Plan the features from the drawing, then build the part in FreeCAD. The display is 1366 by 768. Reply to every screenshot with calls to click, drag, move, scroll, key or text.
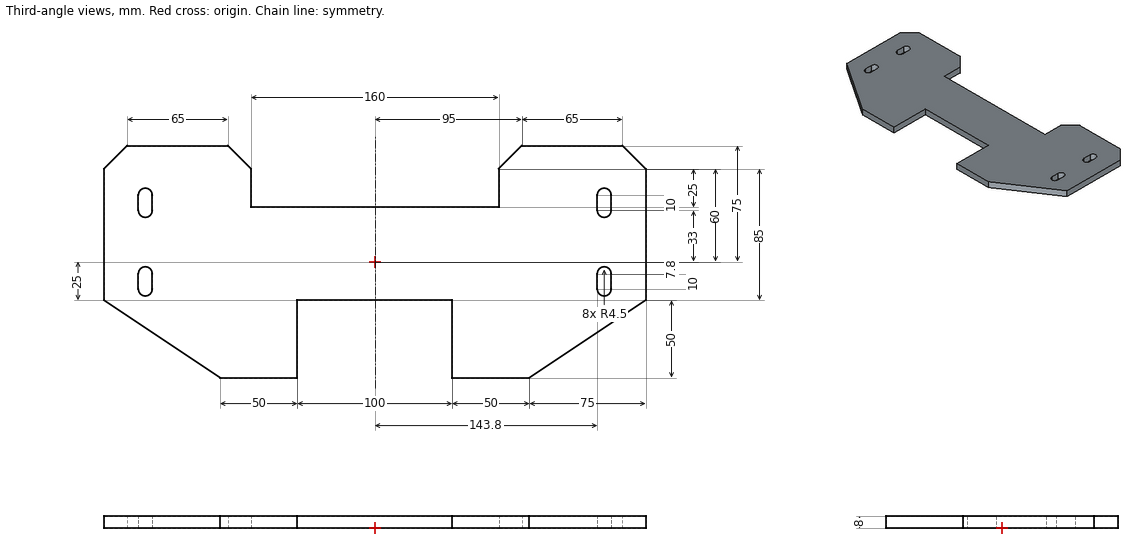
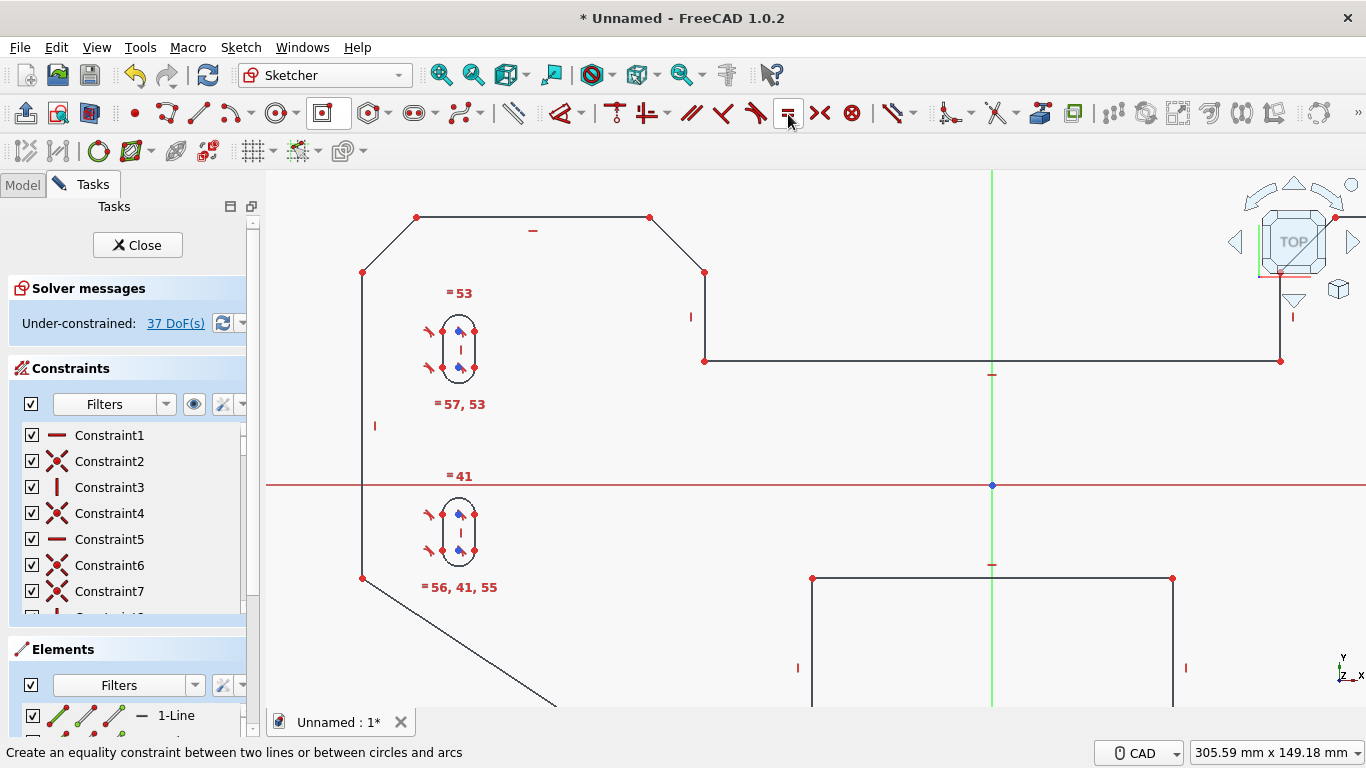
scroll(449, 381, down, 3)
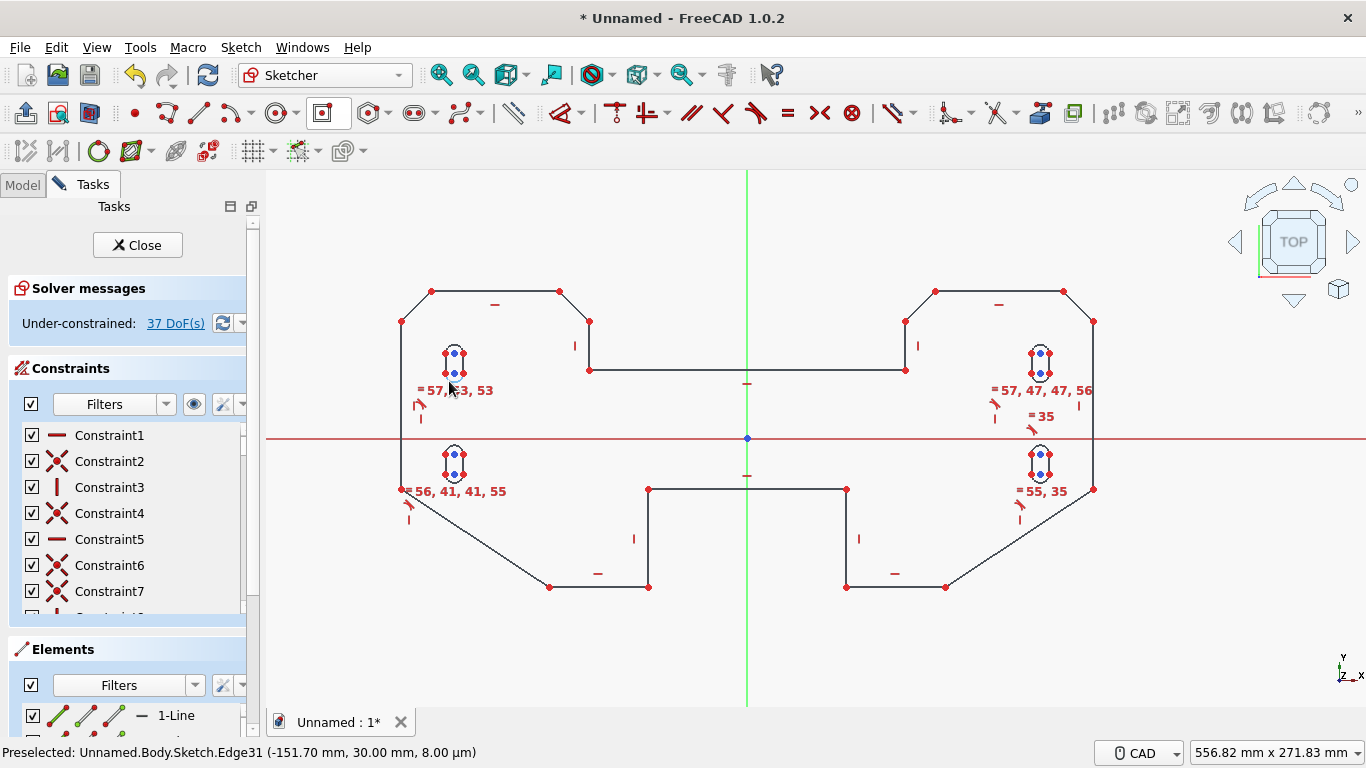
scroll(1040, 474, up, 2)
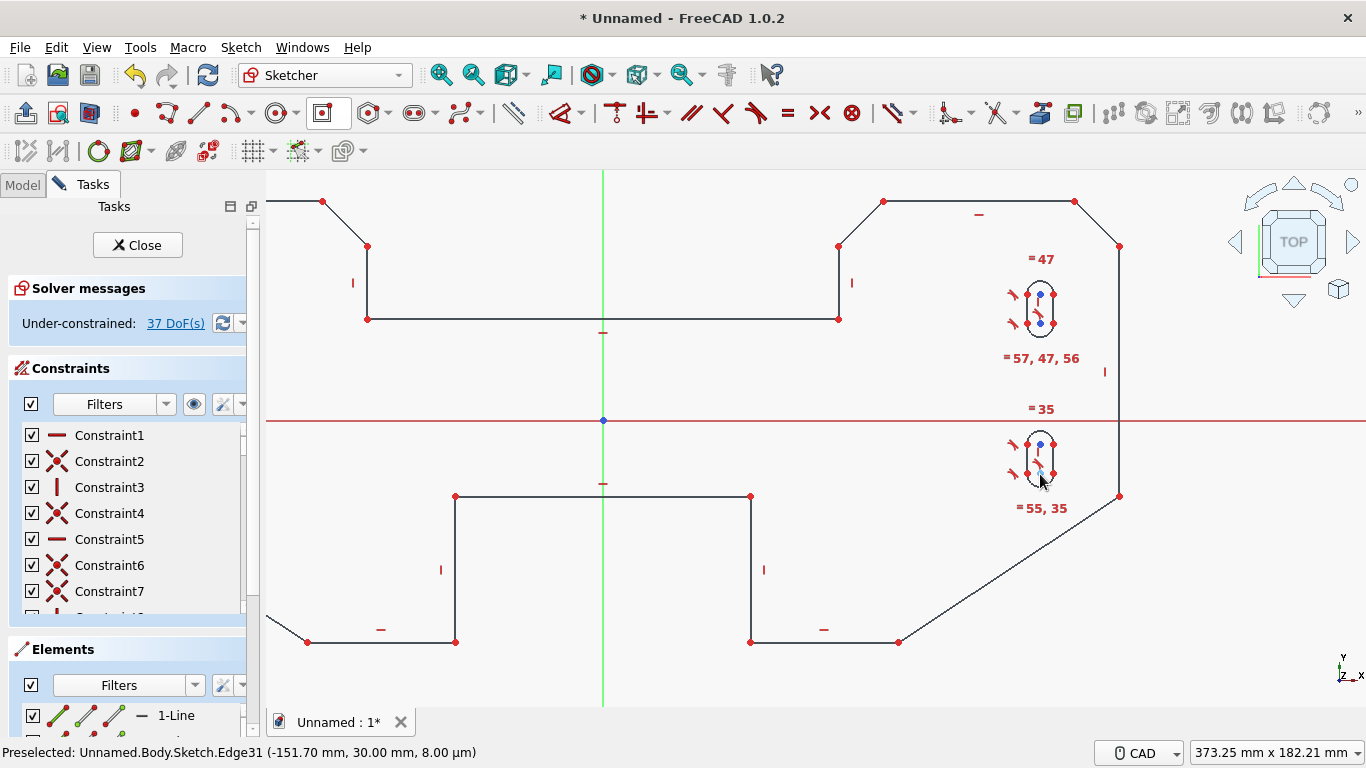
click(1040, 474)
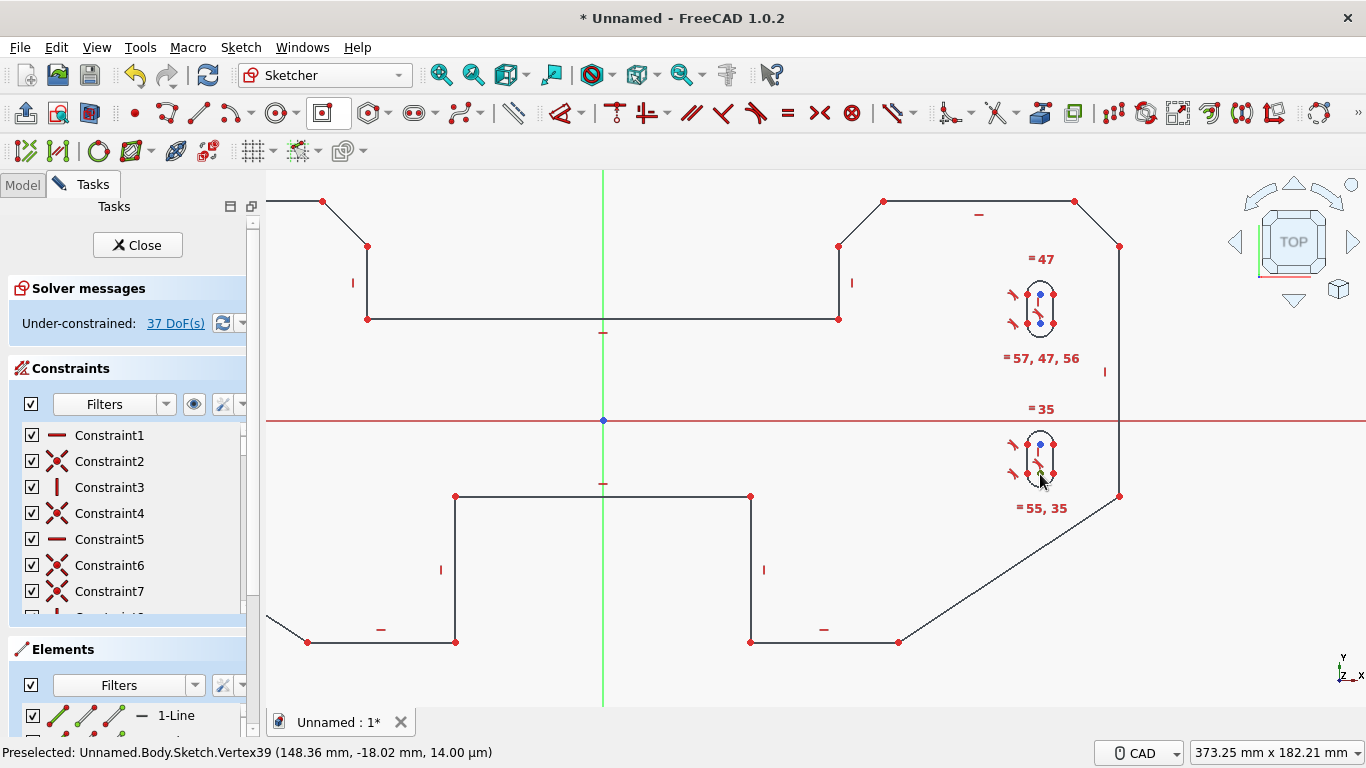
scroll(1041, 475, down, 2)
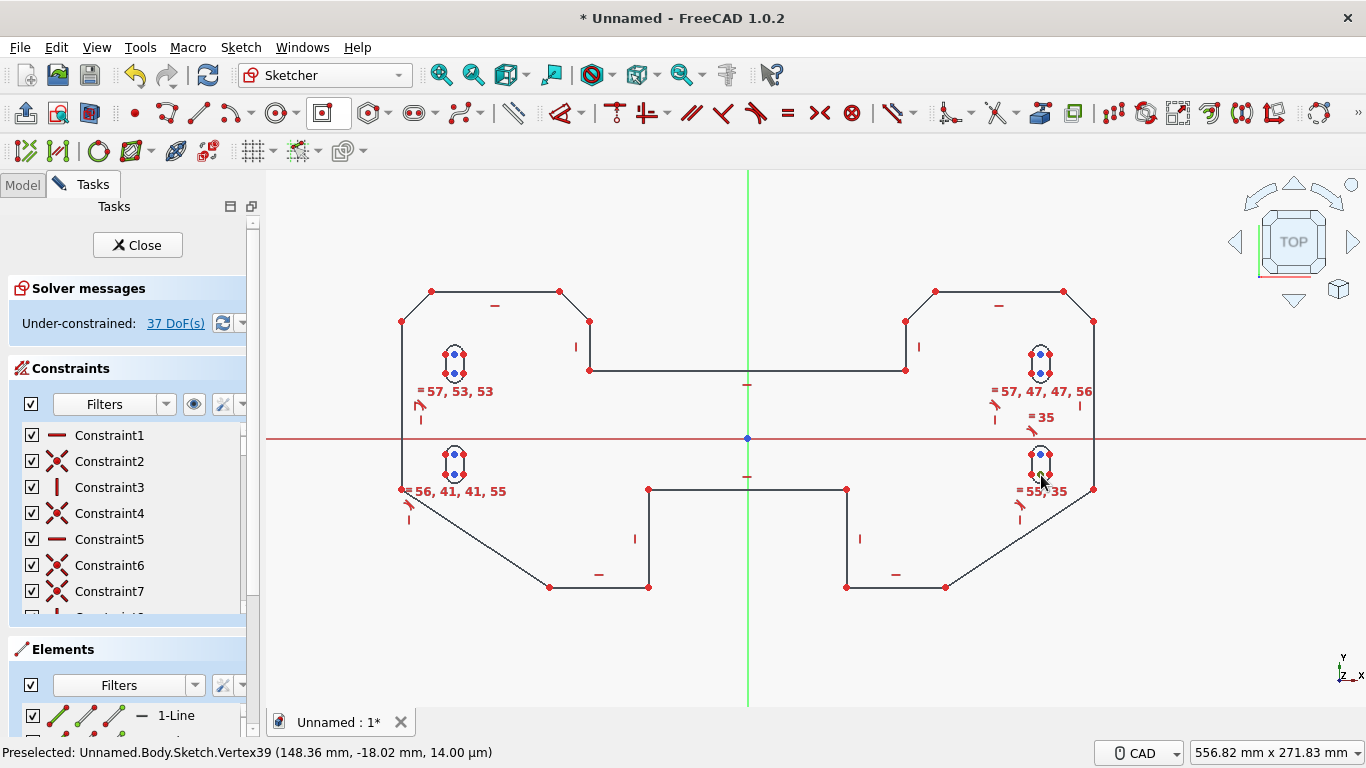
scroll(455, 474, up, 2)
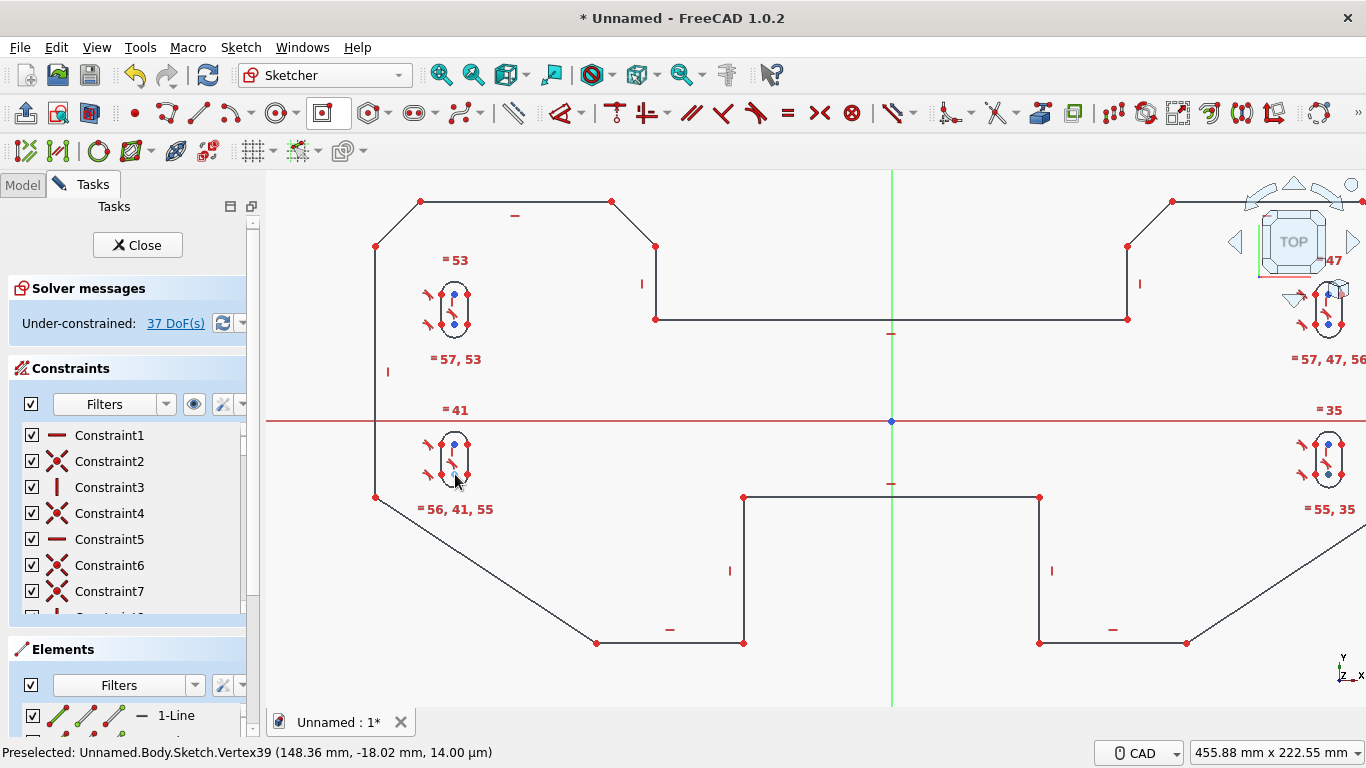
click(455, 474)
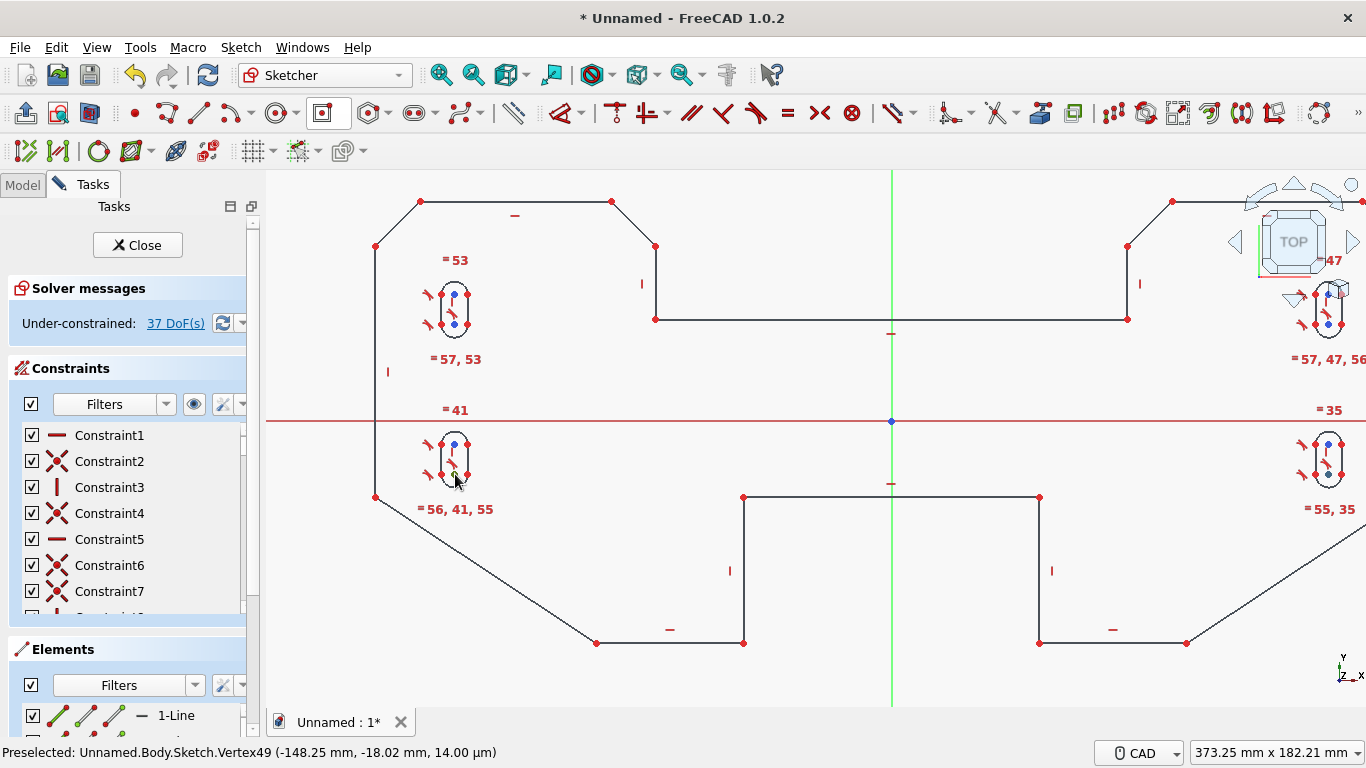
click(892, 645)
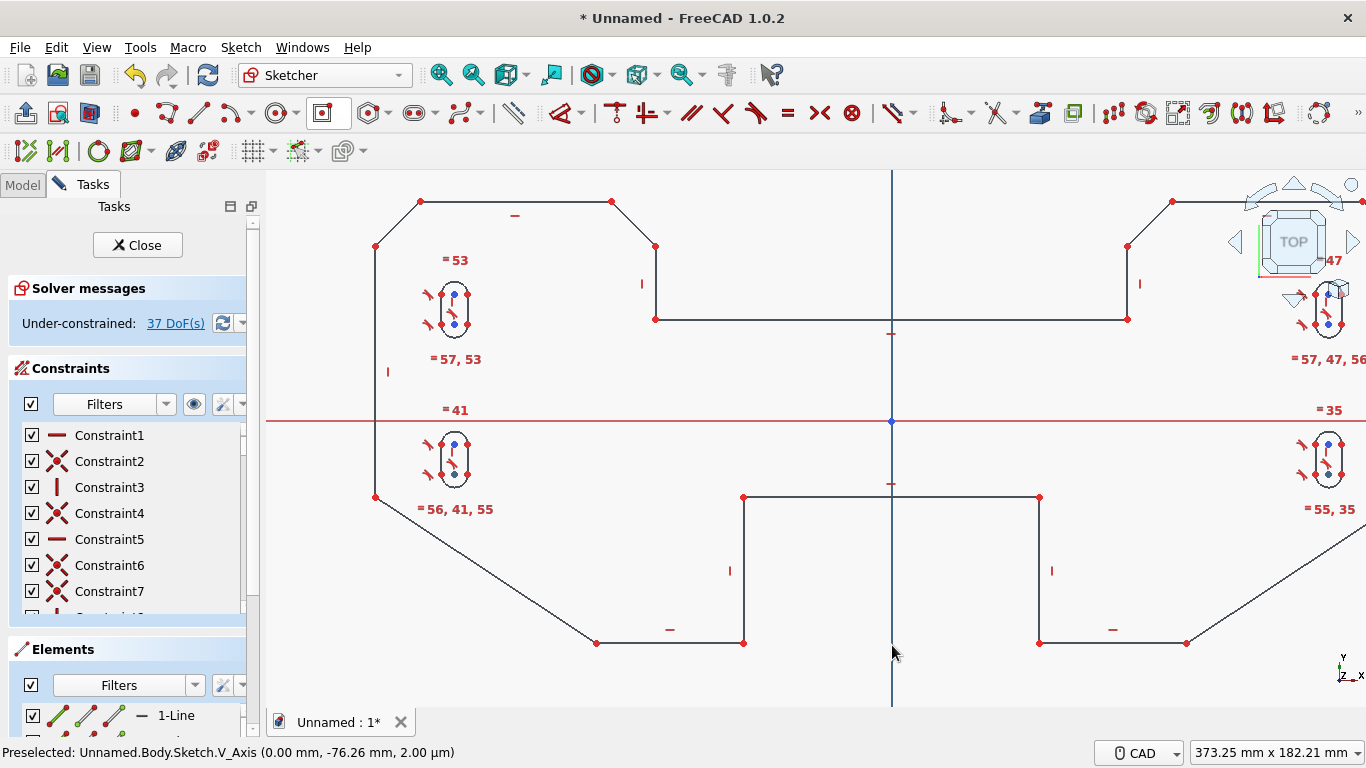
click(820, 114)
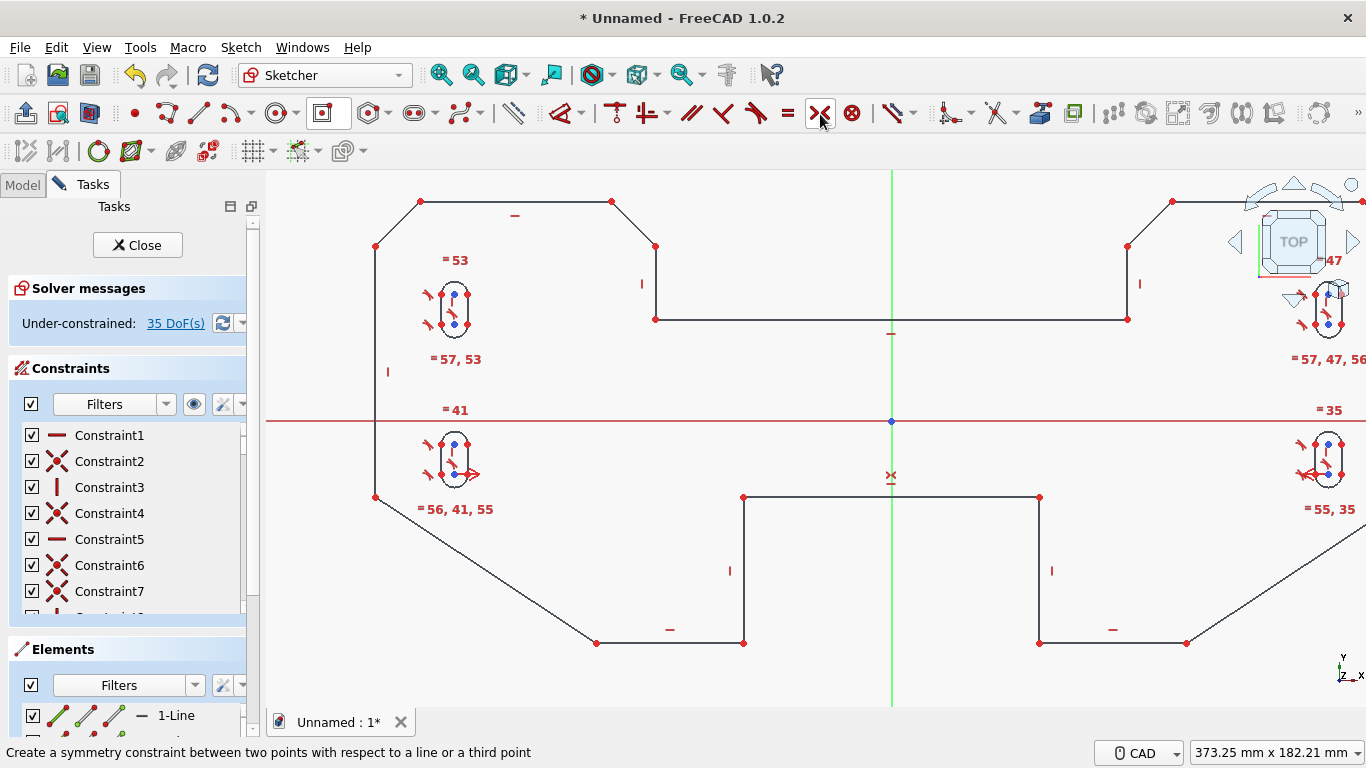
scroll(455, 474, down, 2)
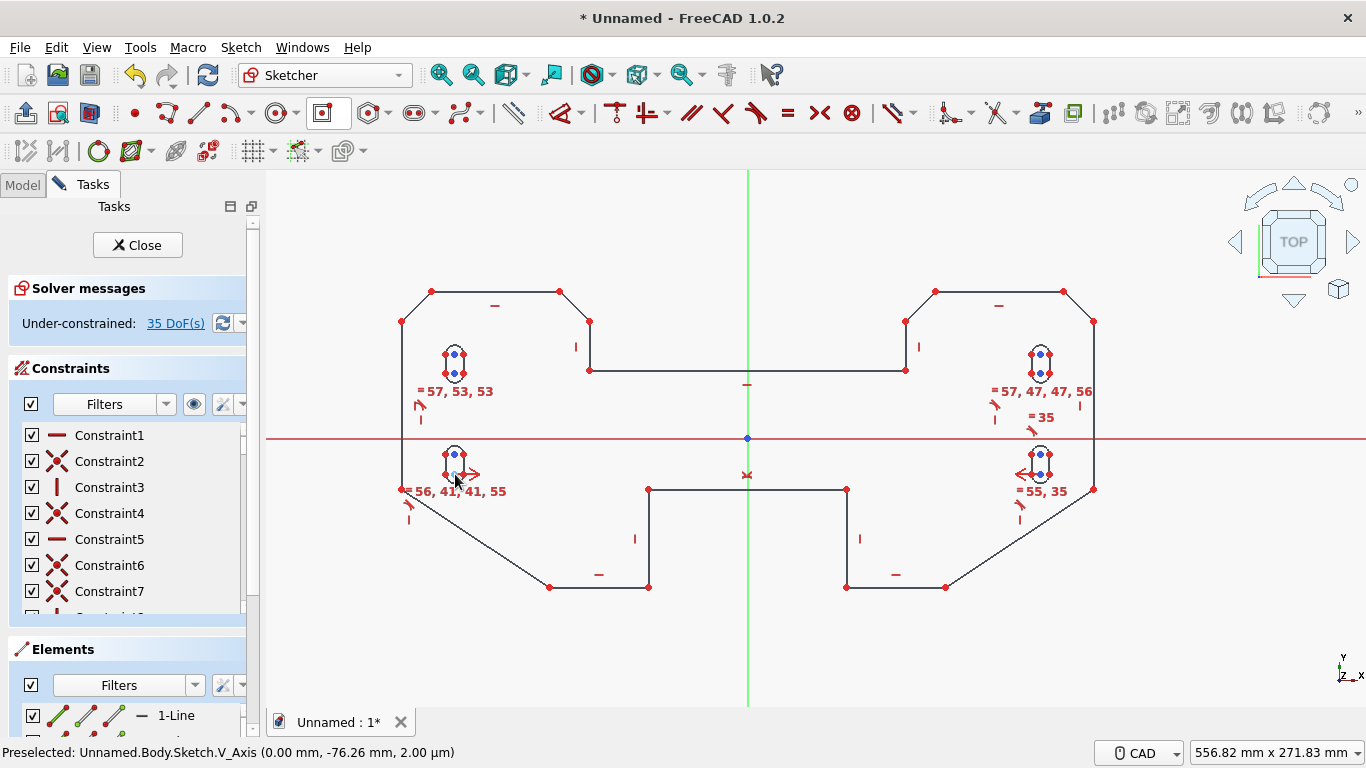
scroll(1041, 374, up, 2)